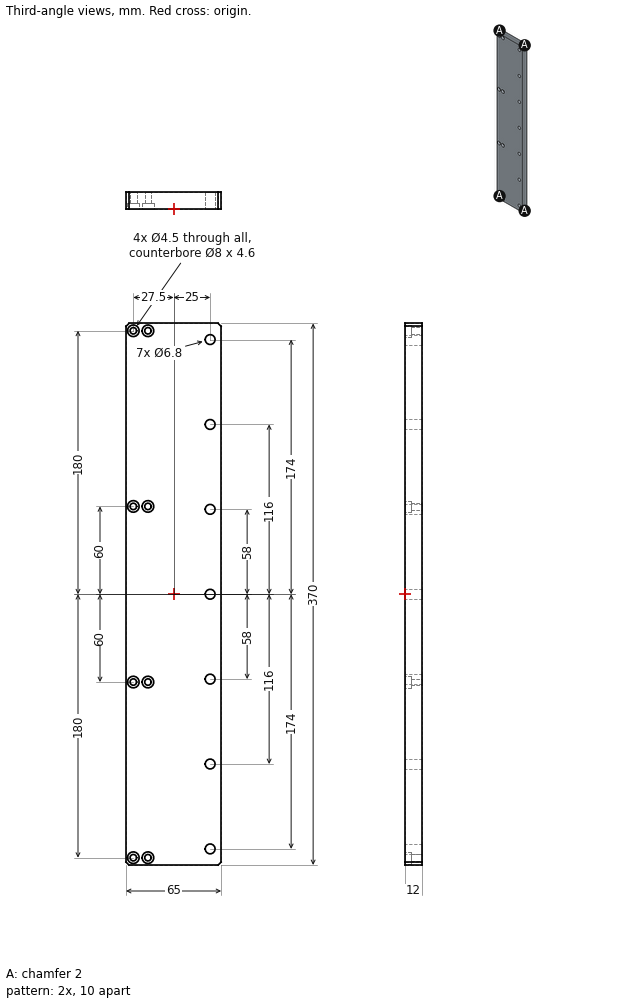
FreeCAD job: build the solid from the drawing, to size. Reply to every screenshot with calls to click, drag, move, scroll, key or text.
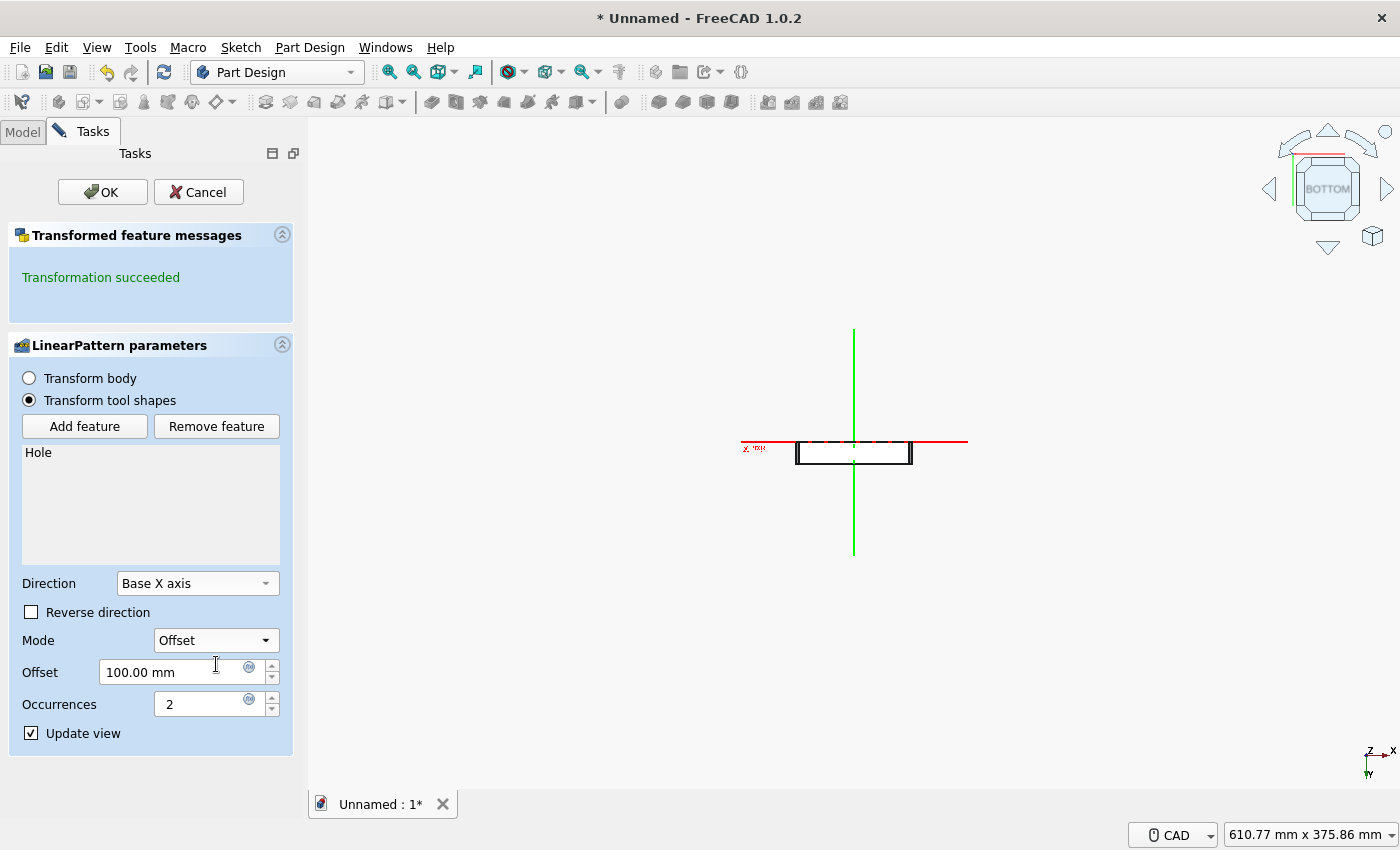
triple_click(182, 672)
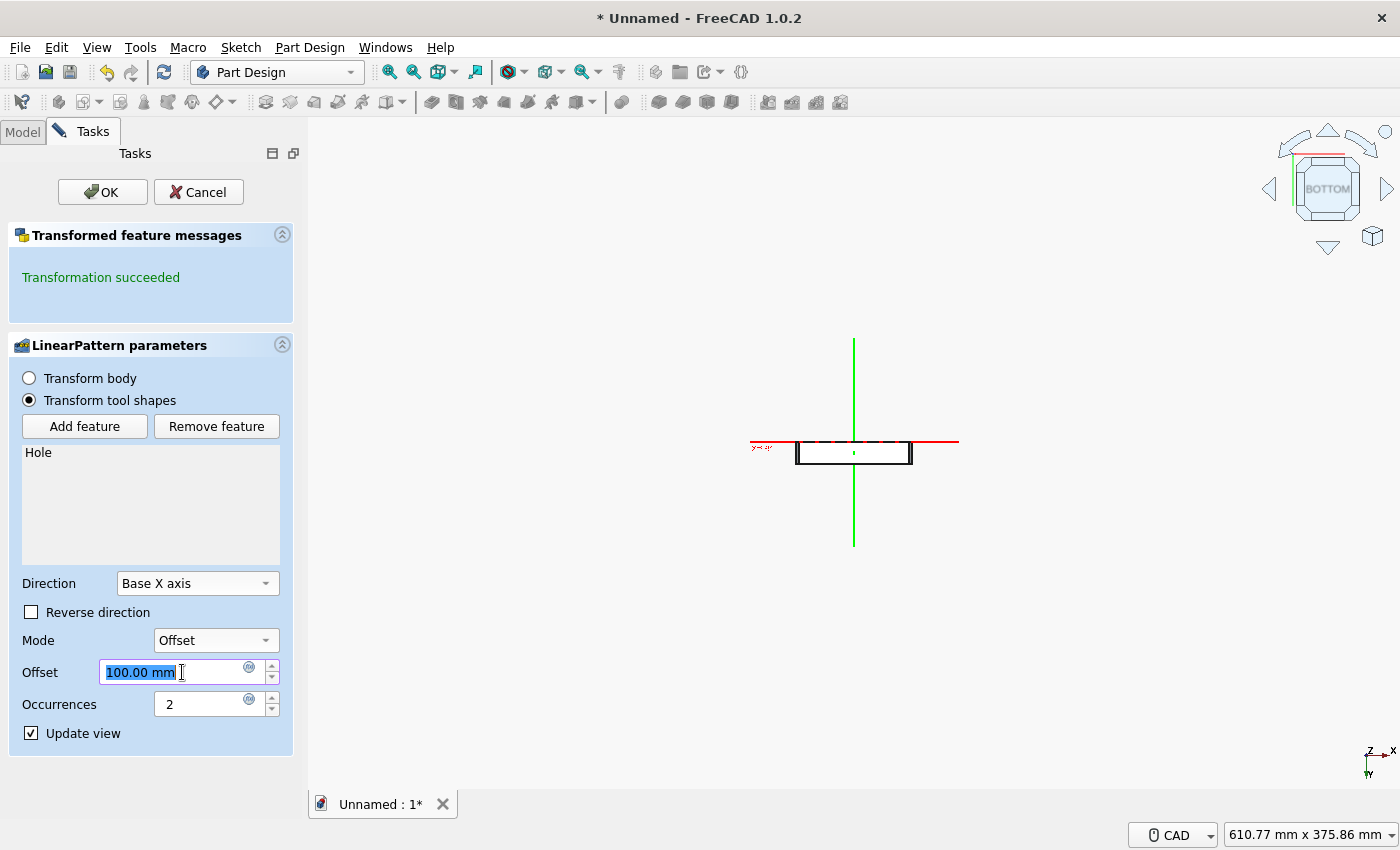
text(10)
key(Tab)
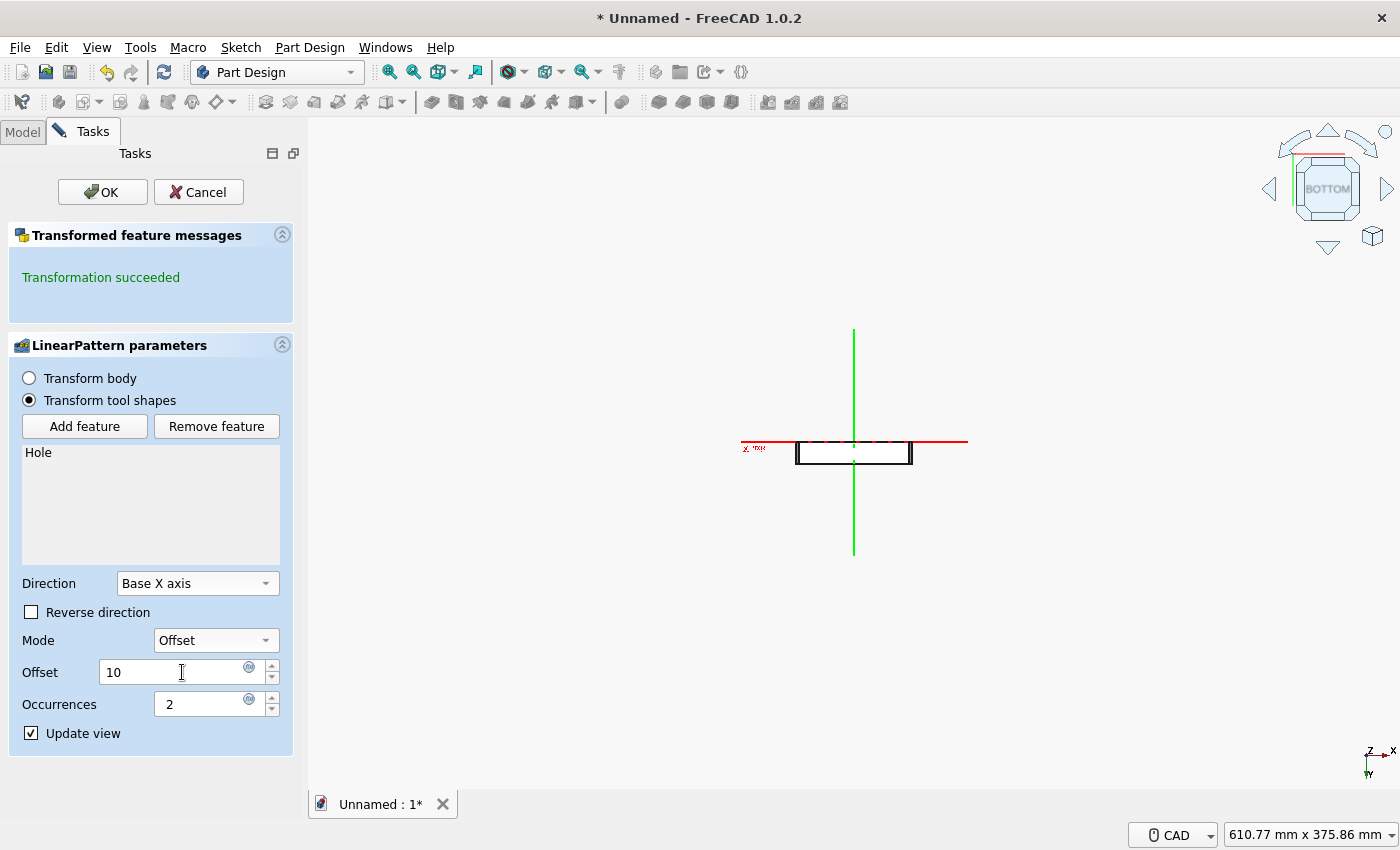
triple_click(209, 704)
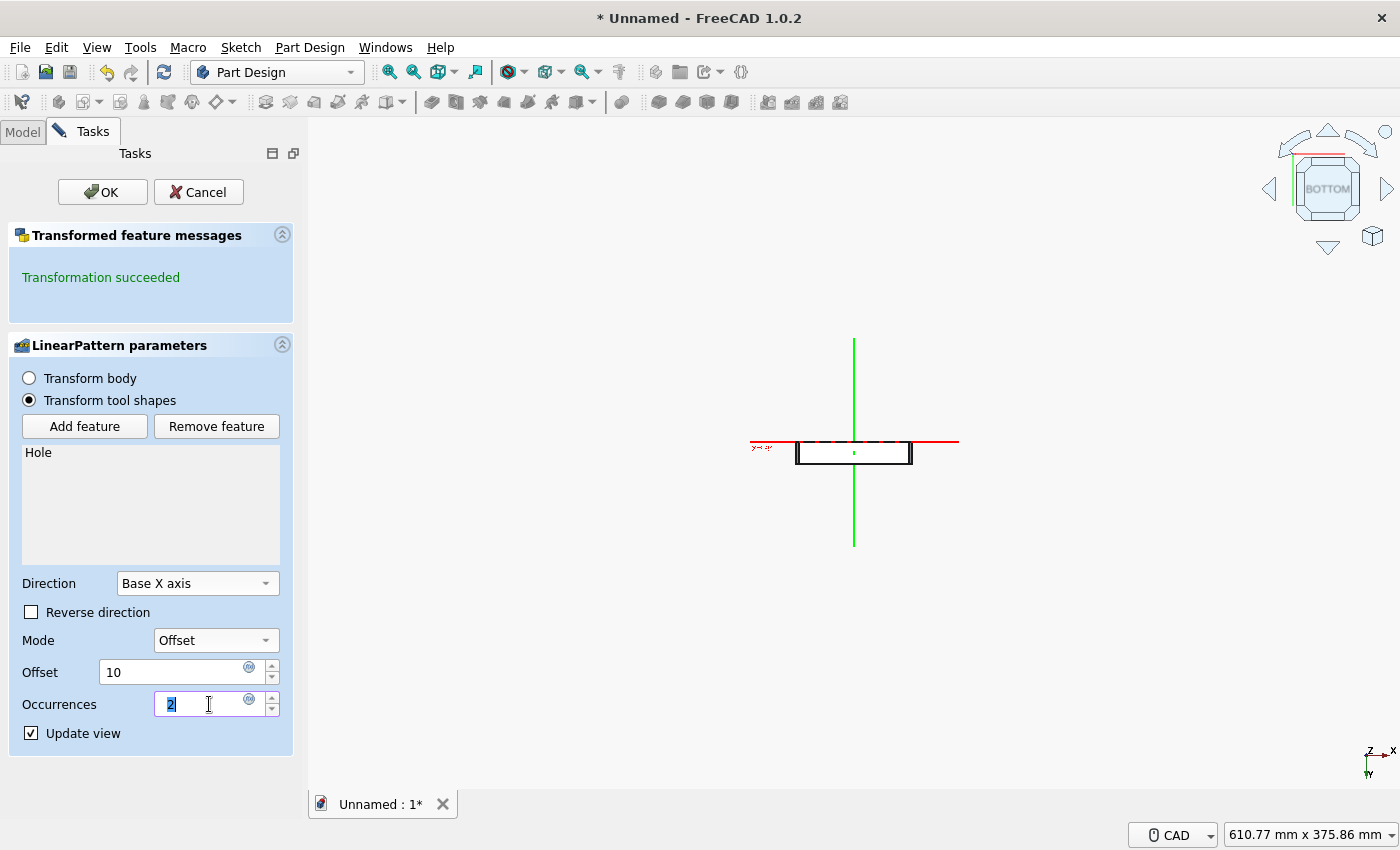
text(2)
key(Tab)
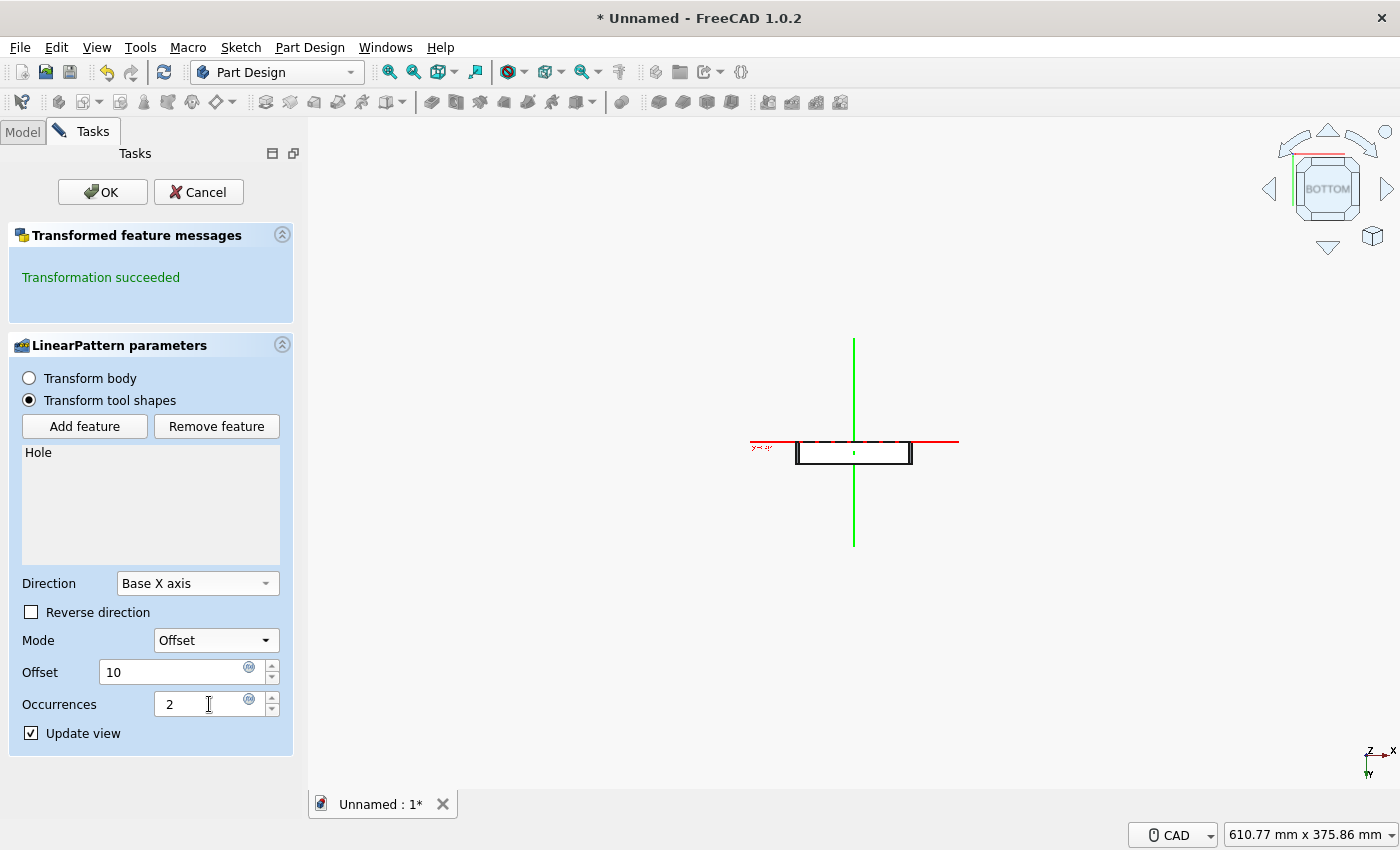
click(103, 192)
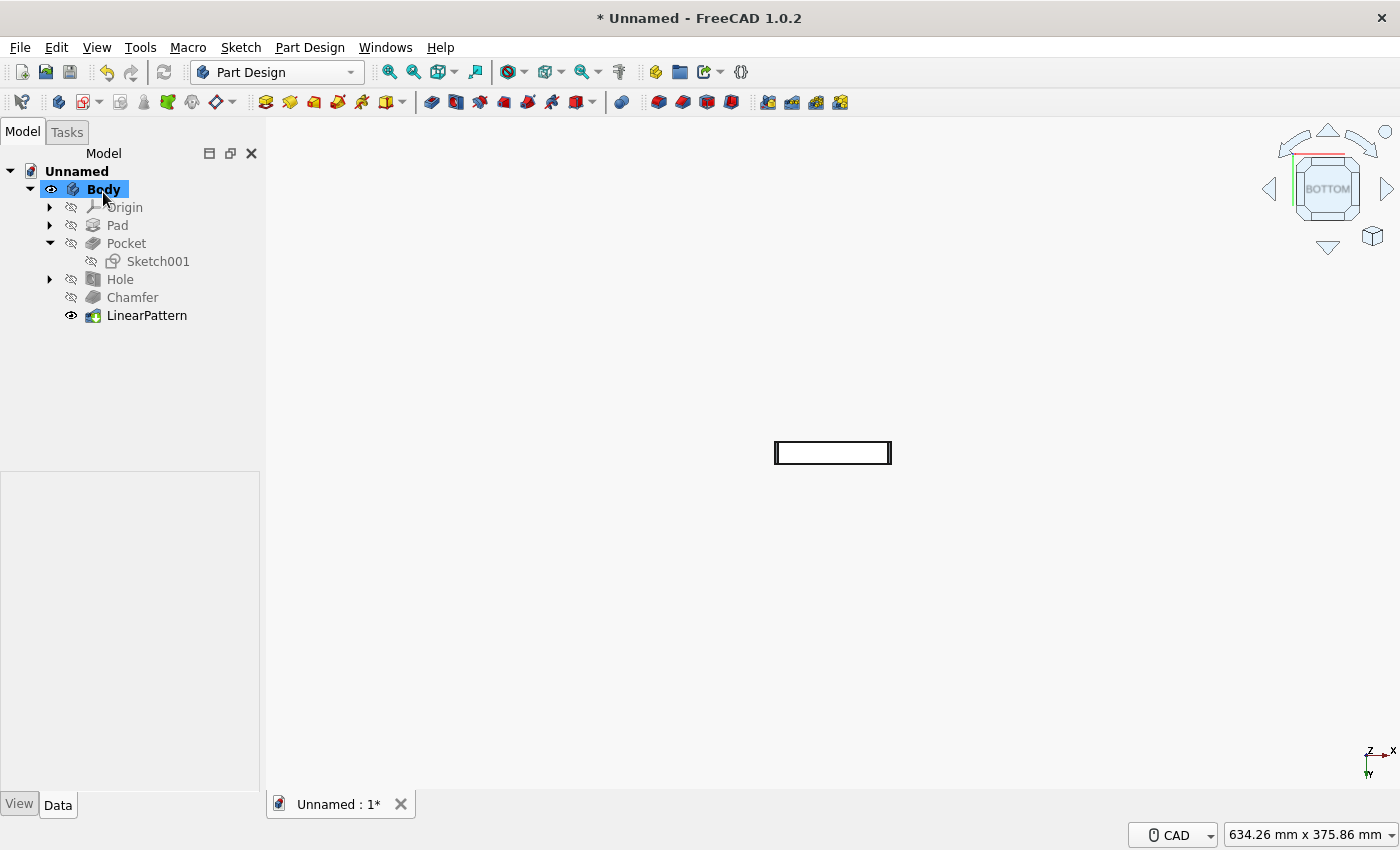
key(0)